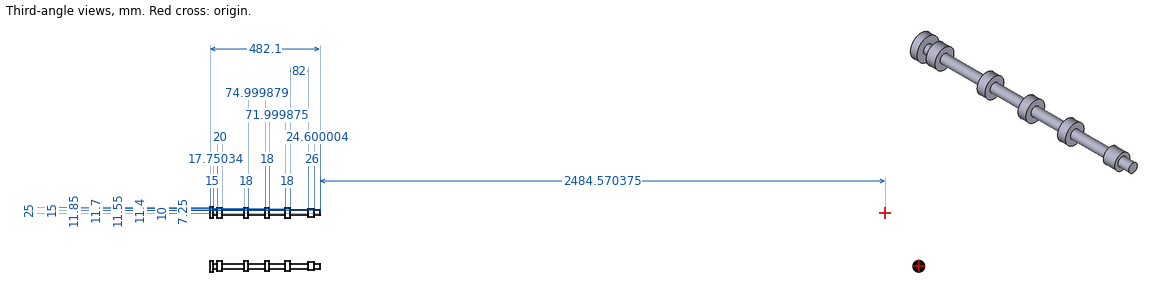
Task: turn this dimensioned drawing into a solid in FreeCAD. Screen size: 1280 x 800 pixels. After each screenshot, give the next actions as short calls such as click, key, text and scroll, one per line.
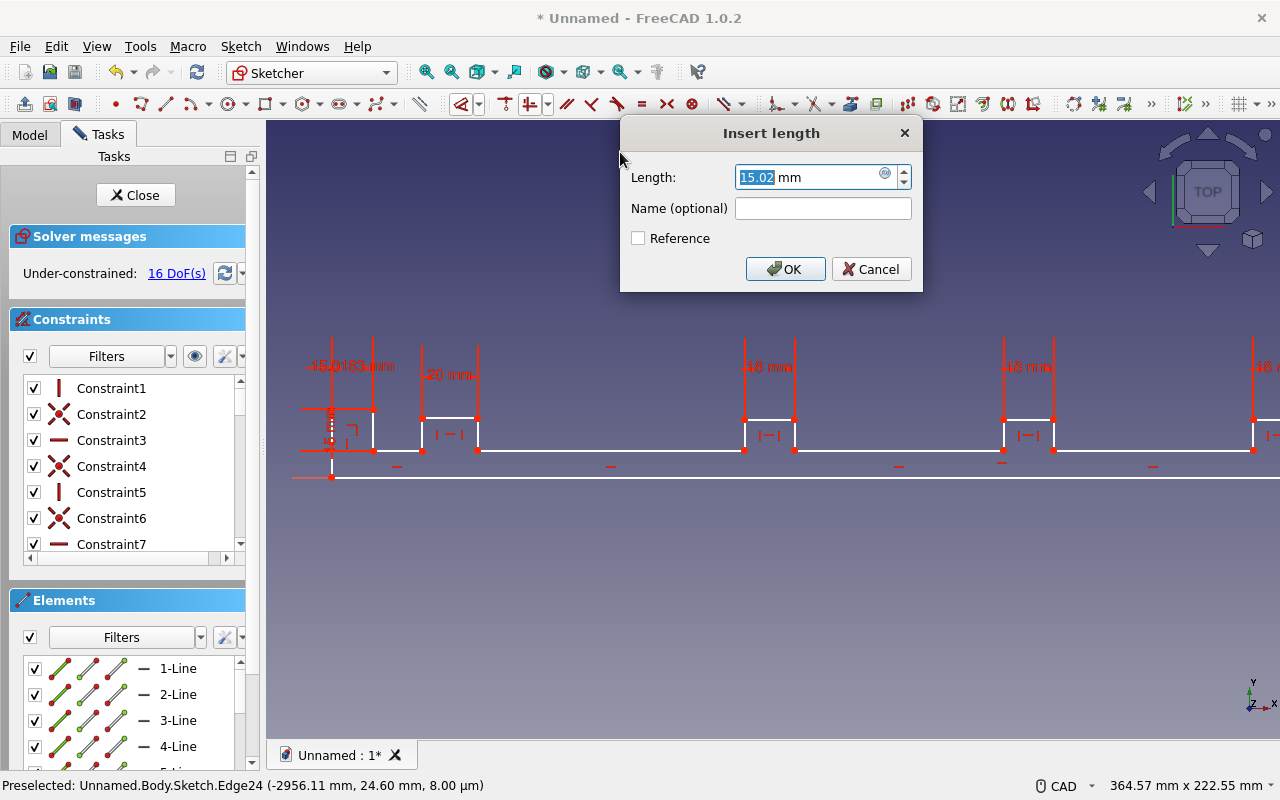
text(15)
key(Return)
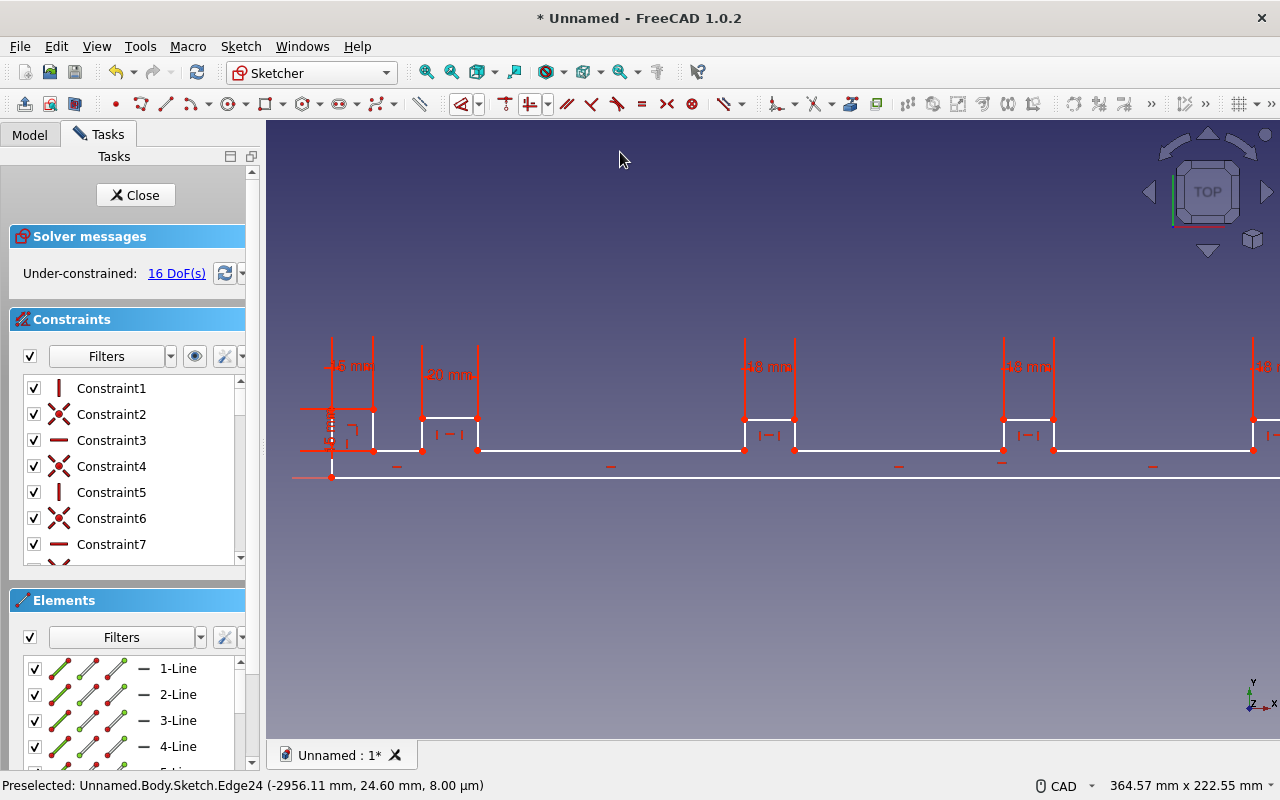
click(332, 457)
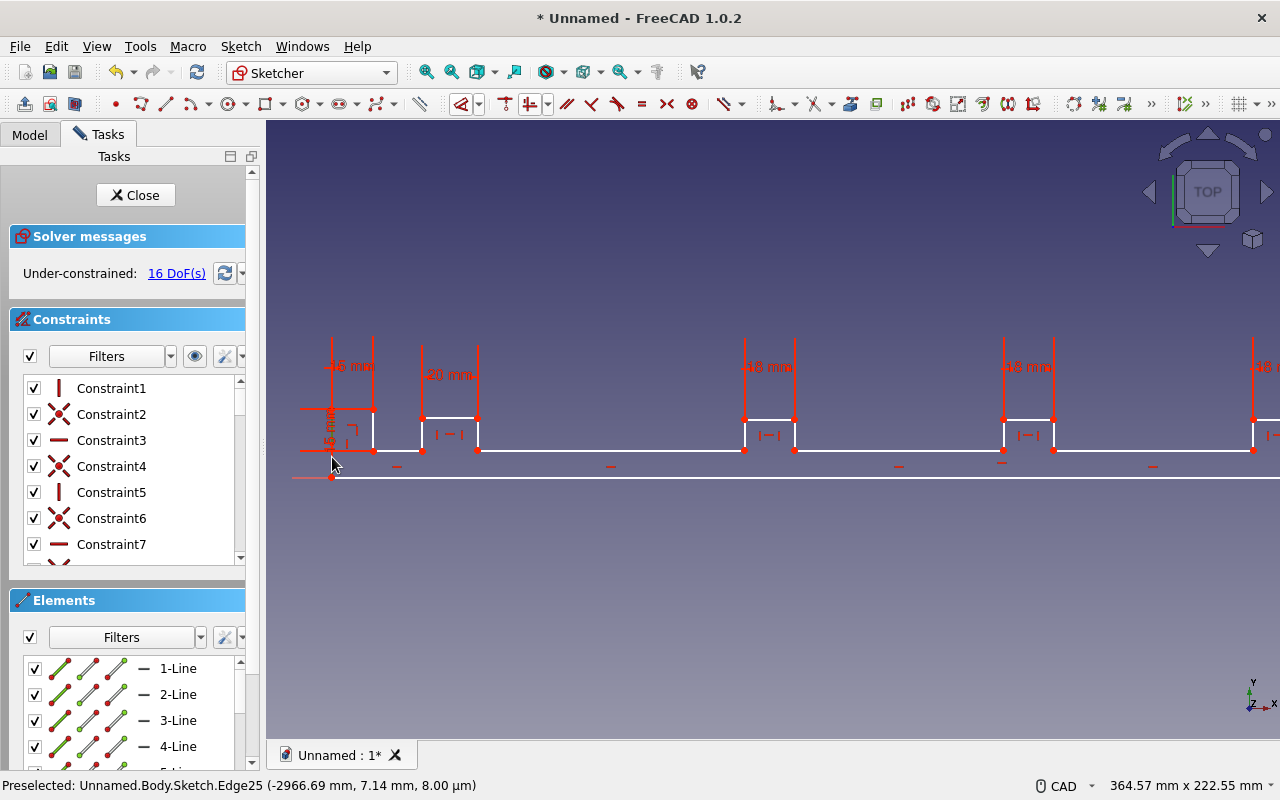
key(i)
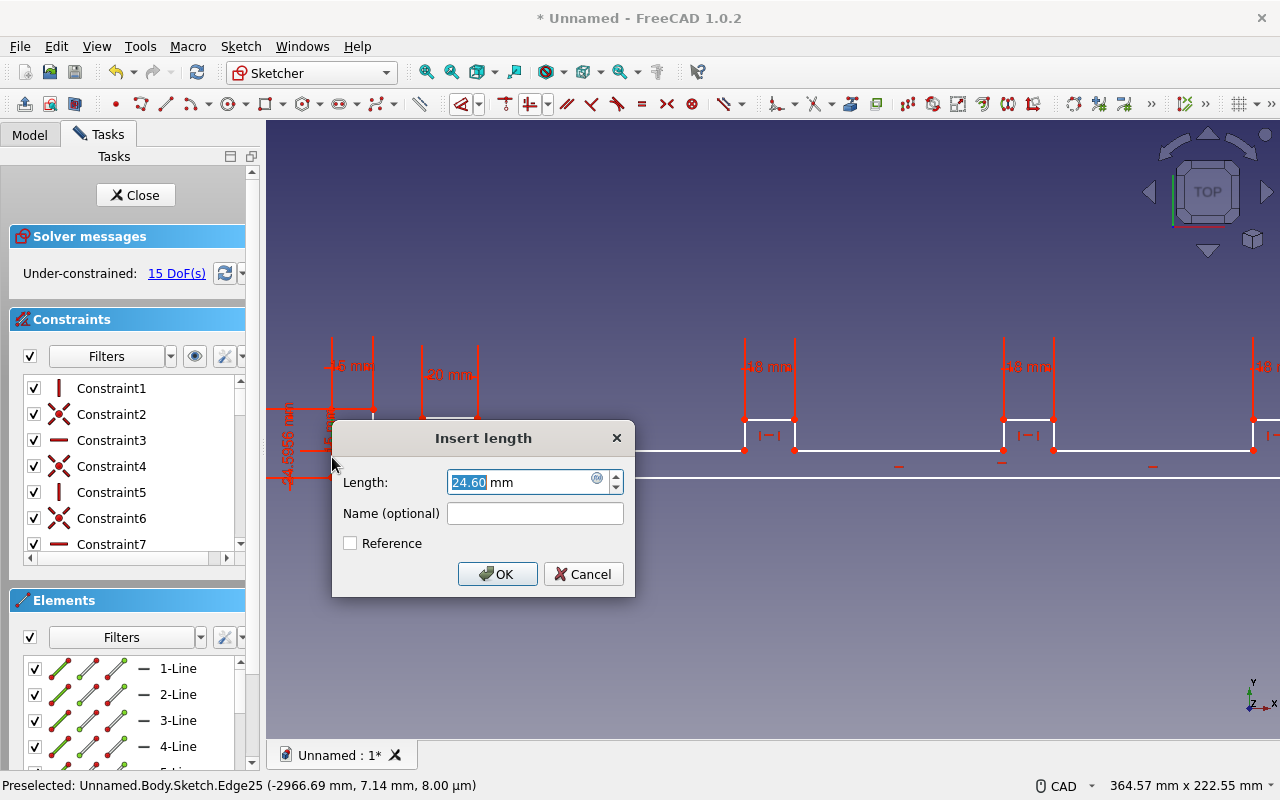
text(25)
key(Return)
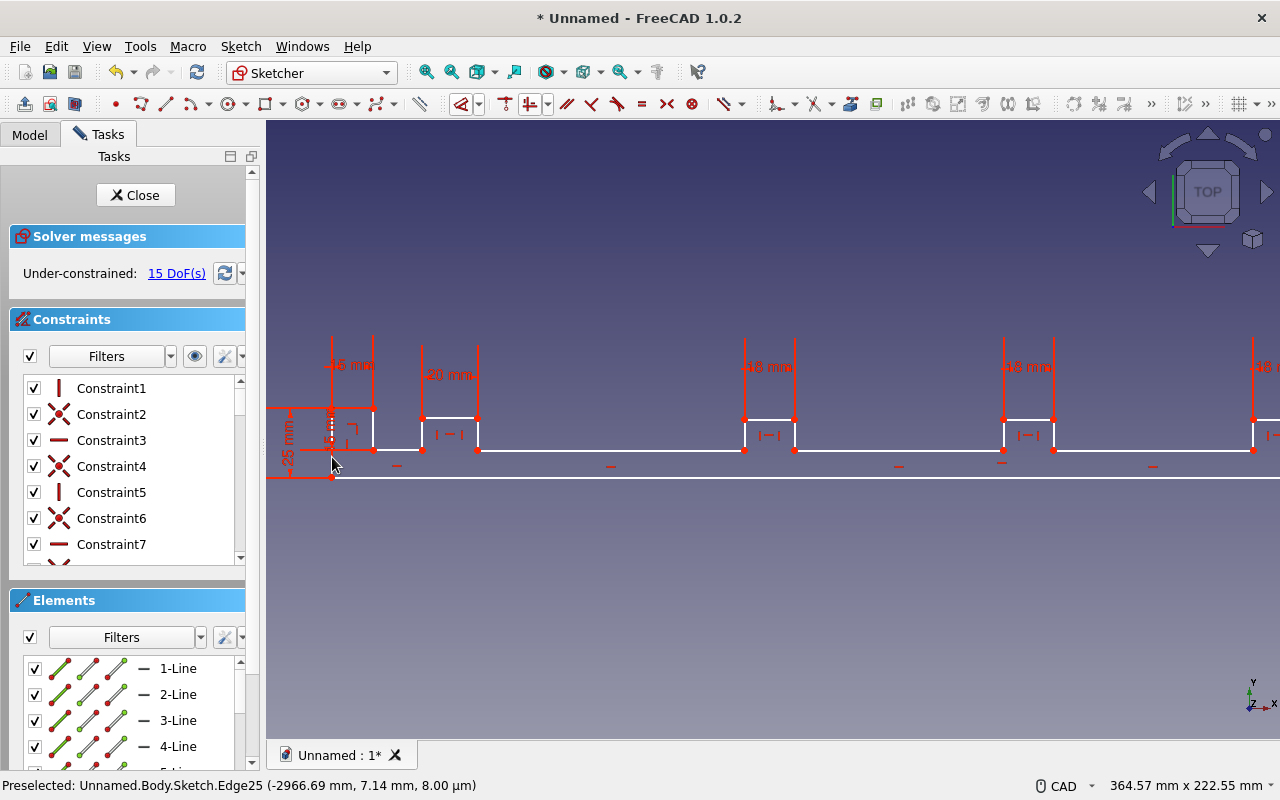
scroll(462, 418, down, 4)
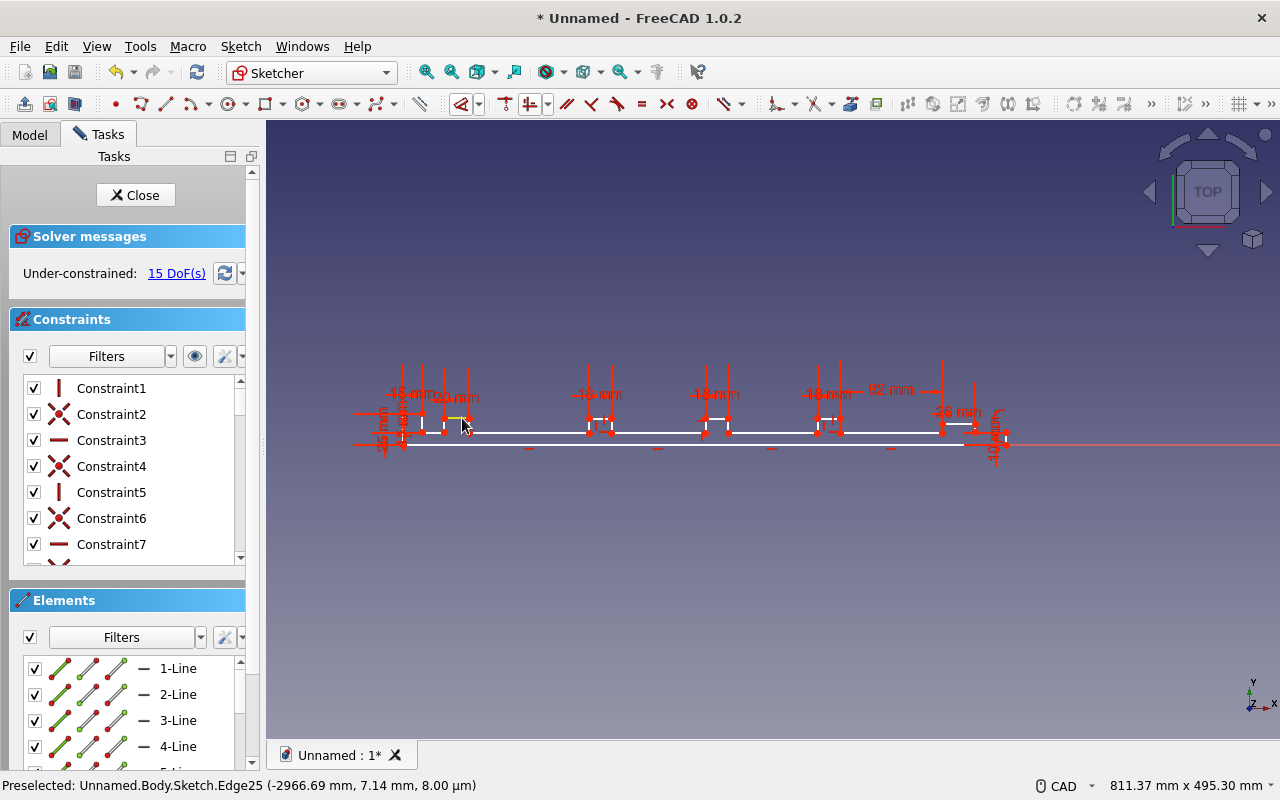
scroll(943, 433, up, 6)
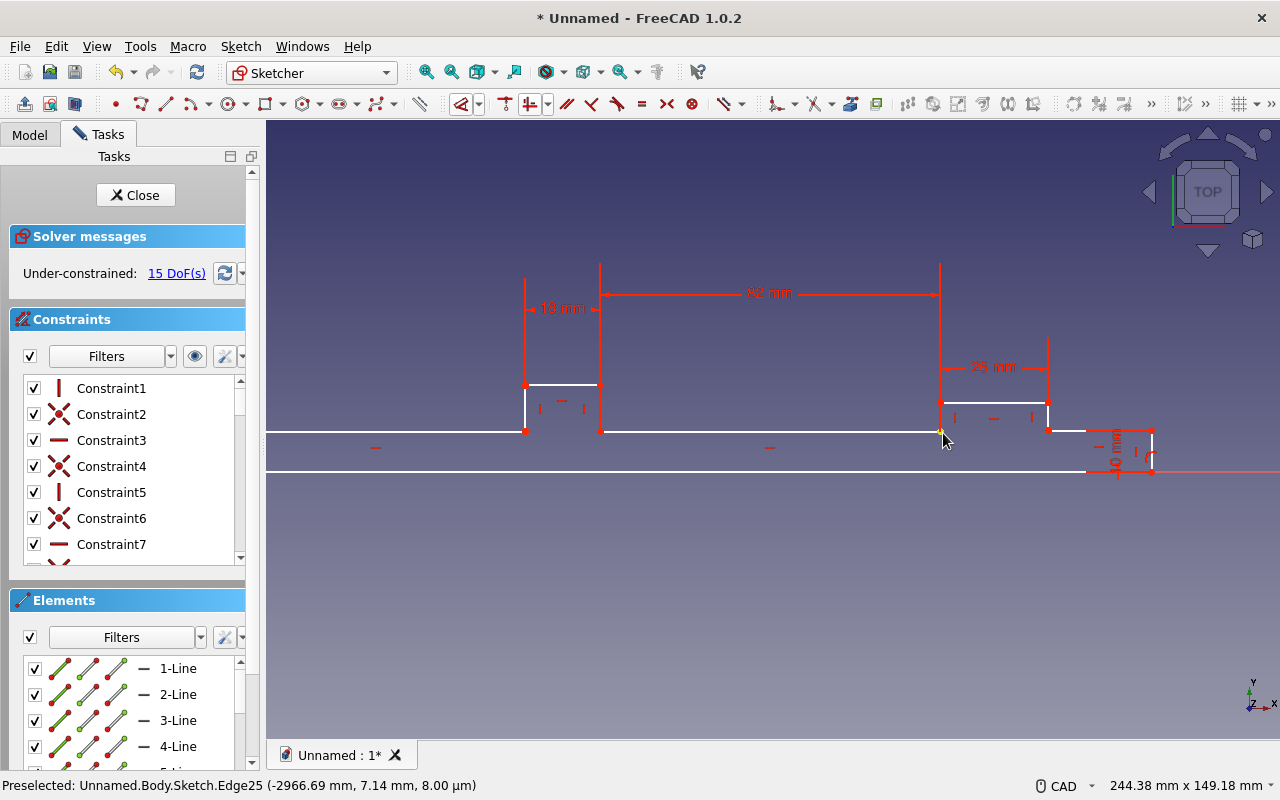
click(940, 432)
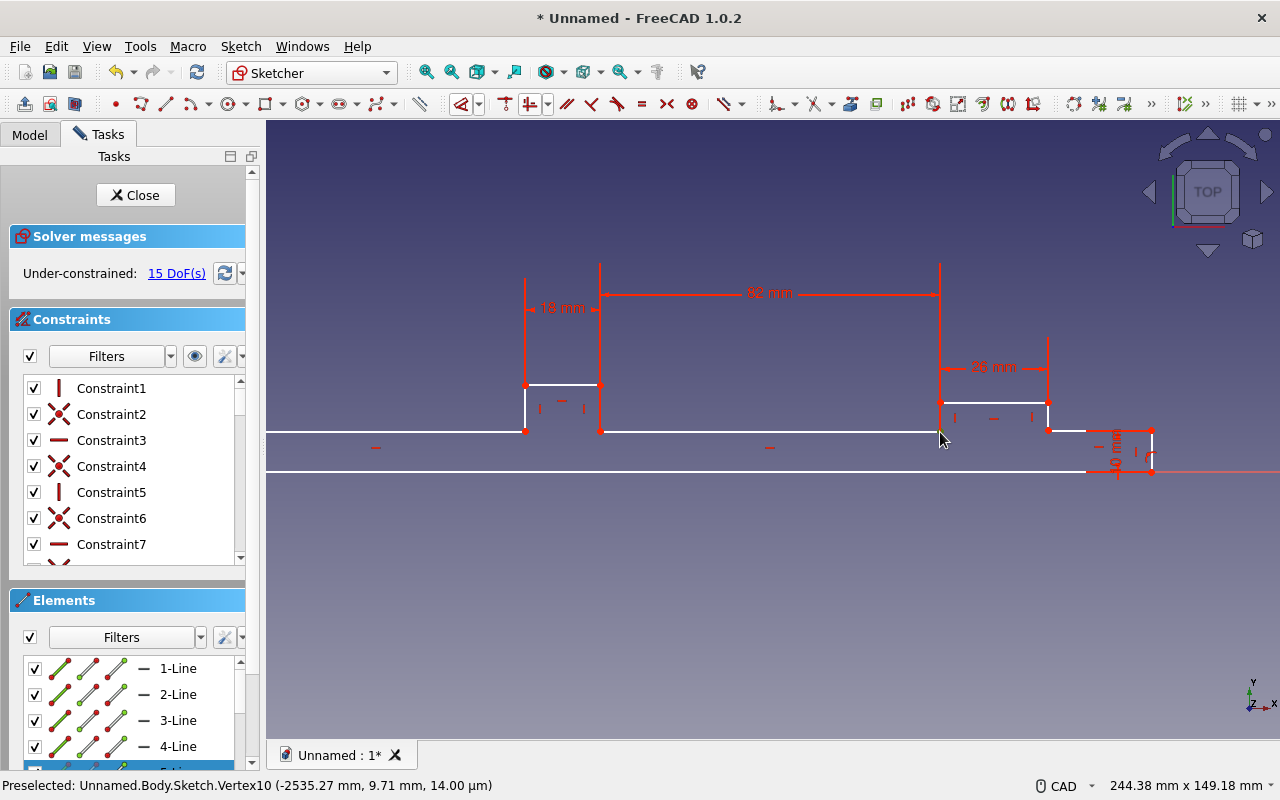
click(478, 104)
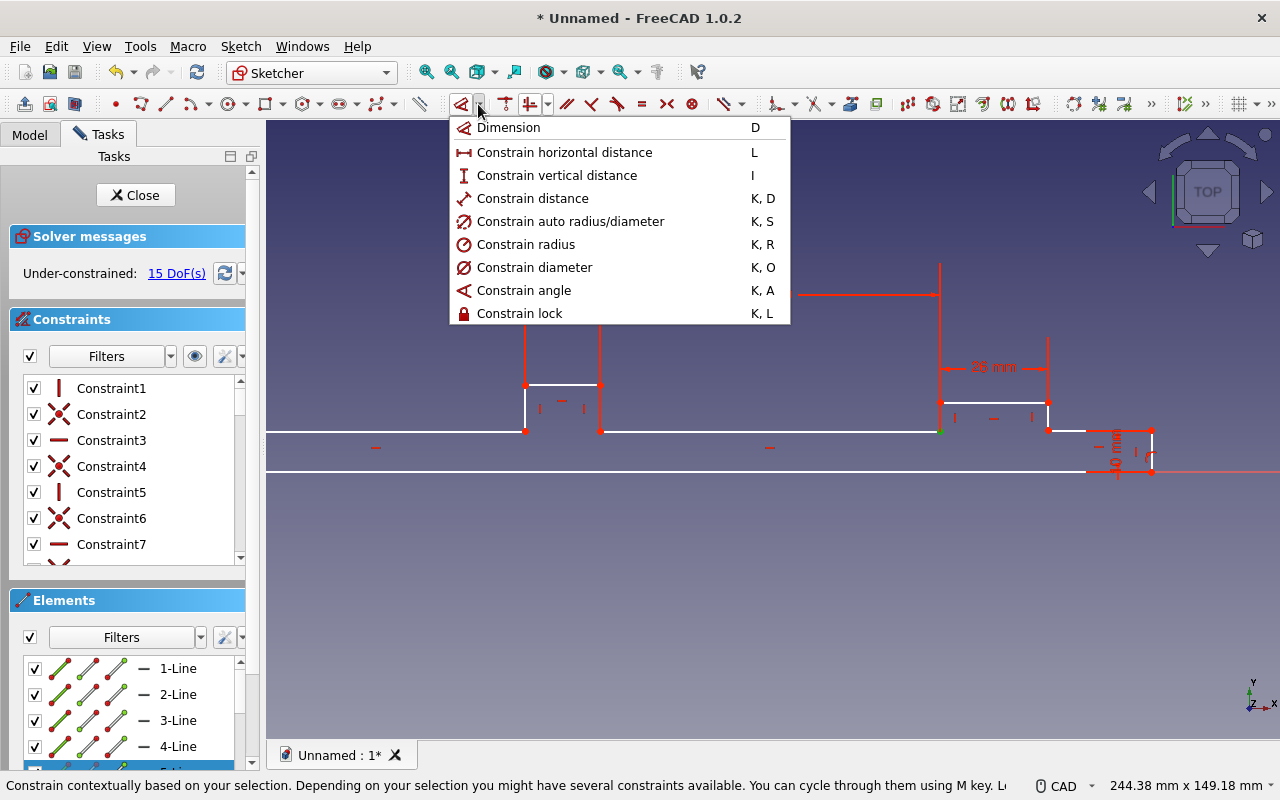
click(620, 176)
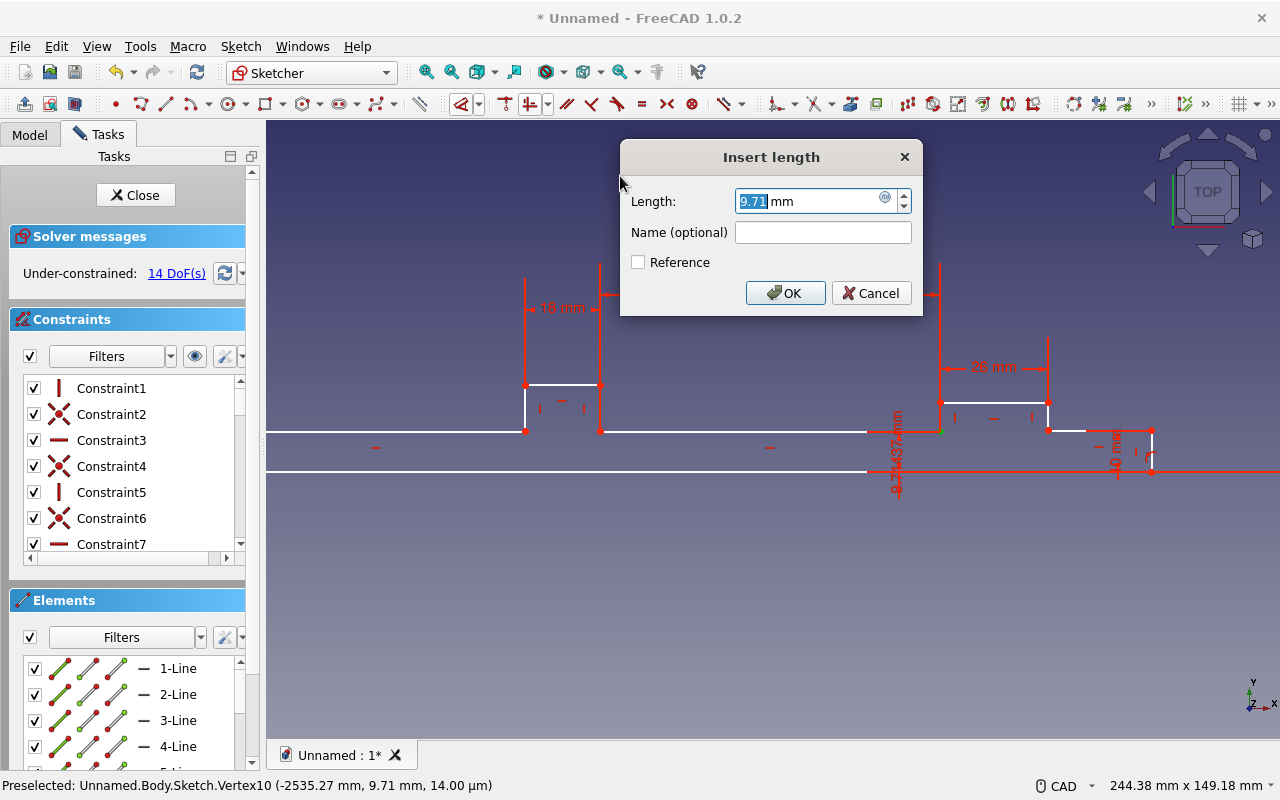
text(10)
key(Return)